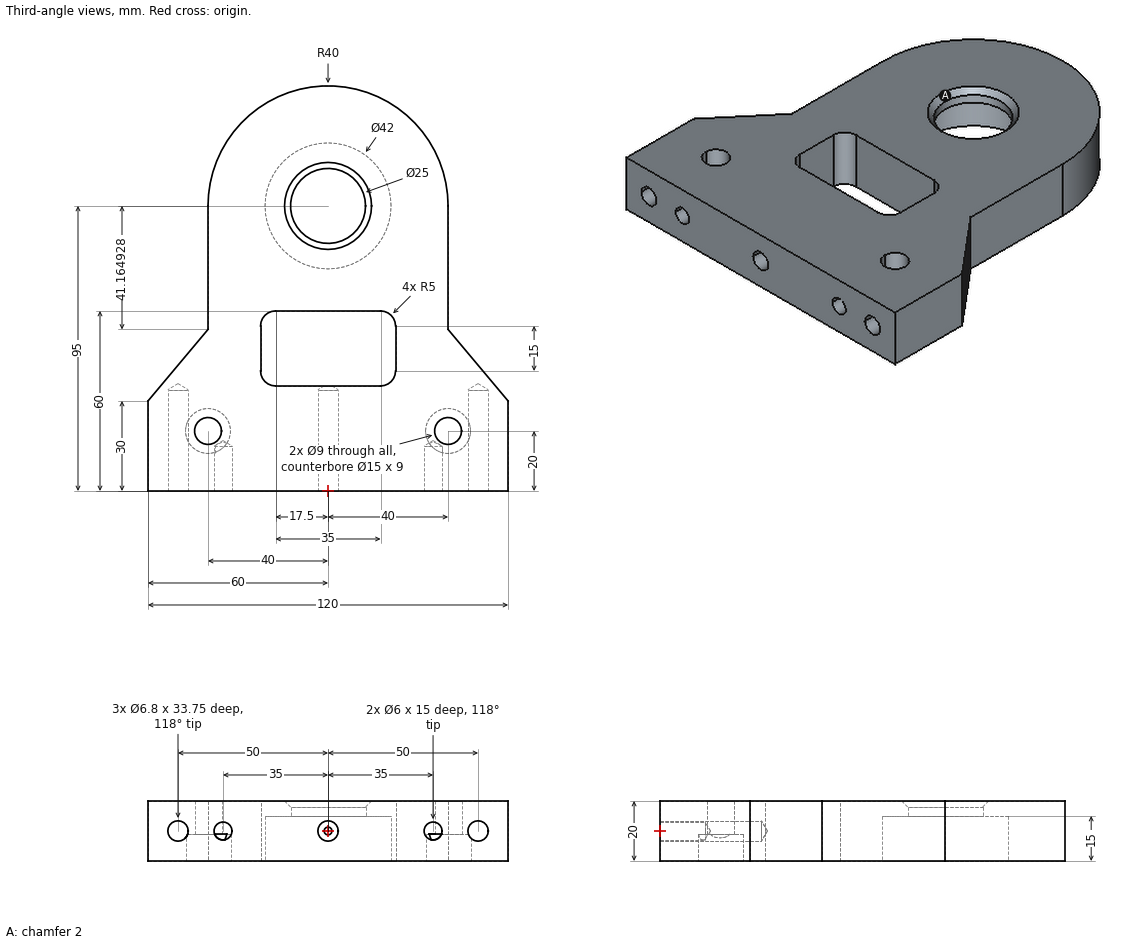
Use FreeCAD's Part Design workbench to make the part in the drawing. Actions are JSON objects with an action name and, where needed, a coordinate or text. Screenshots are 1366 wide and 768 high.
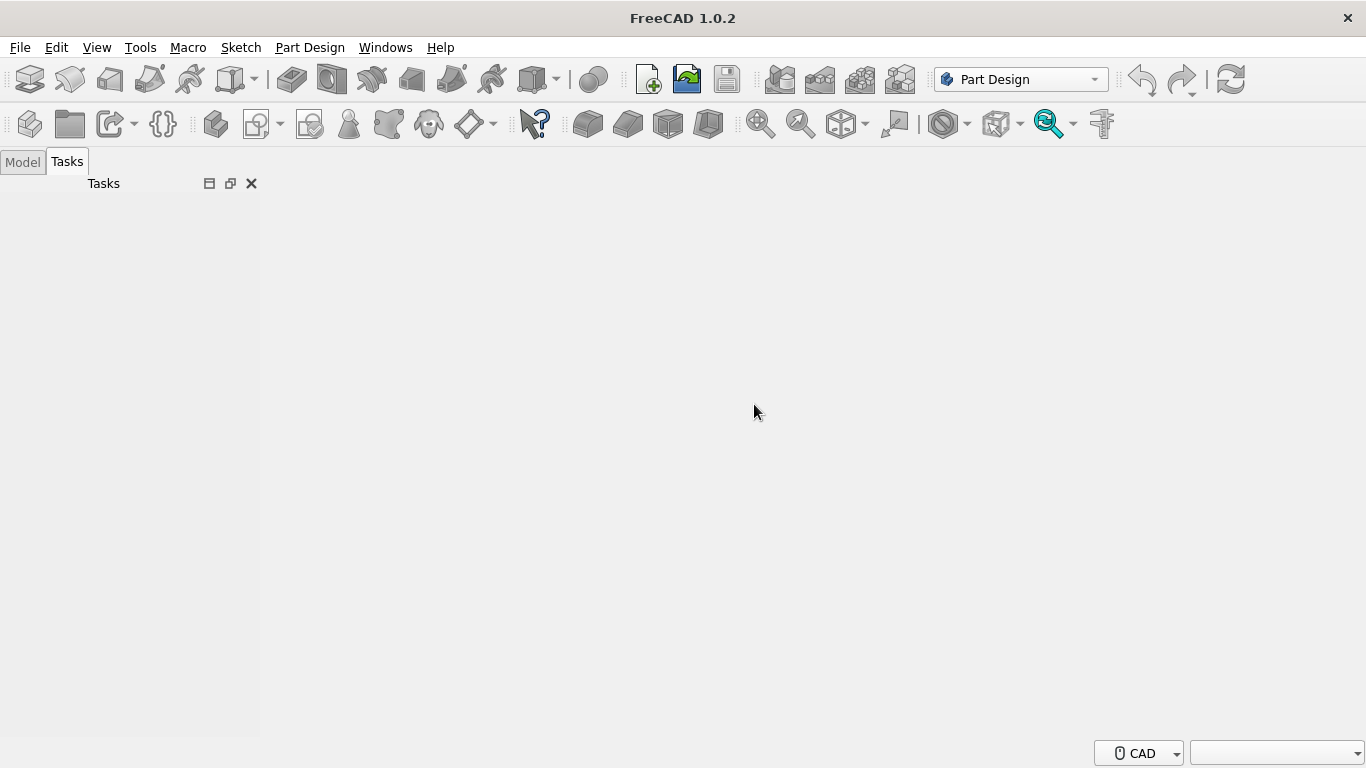
{"action": "left_click", "coordinate": [648, 80]}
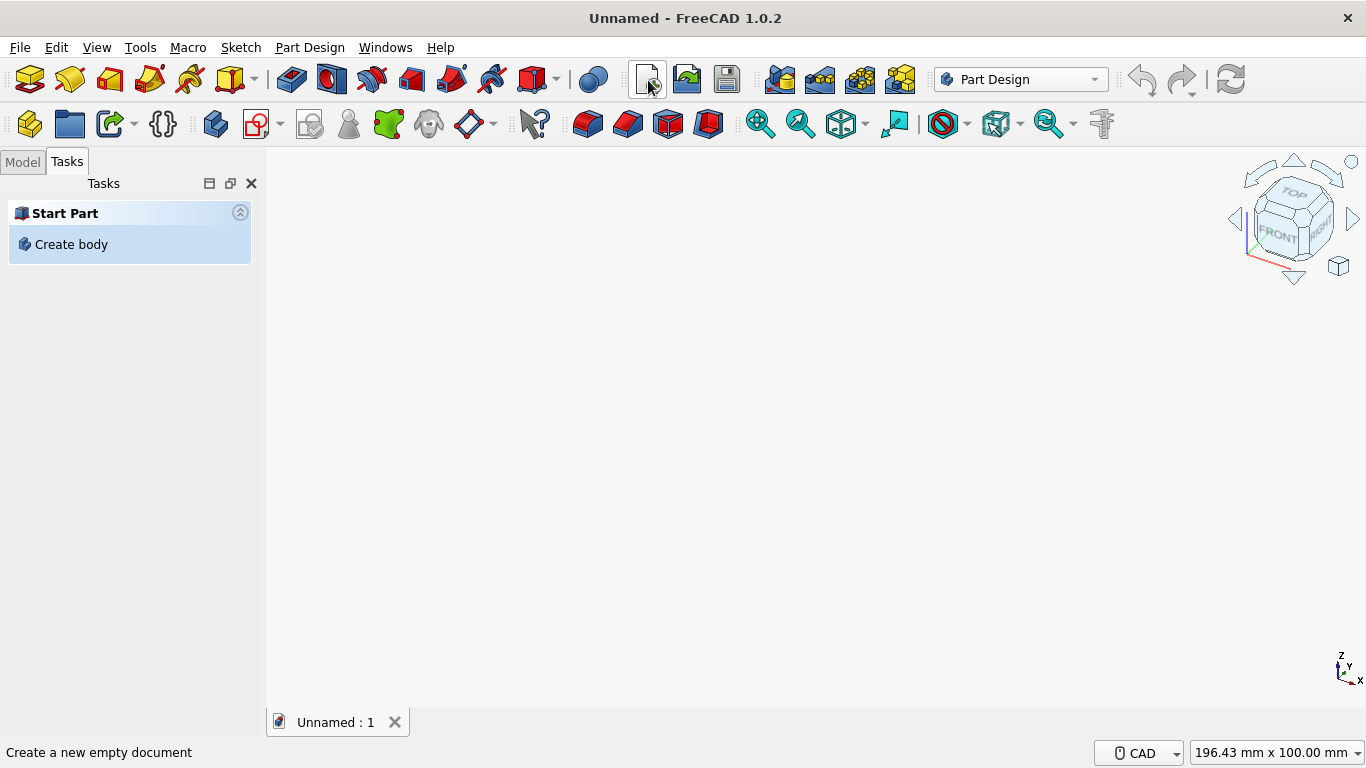
{"action": "left_click", "coordinate": [256, 124]}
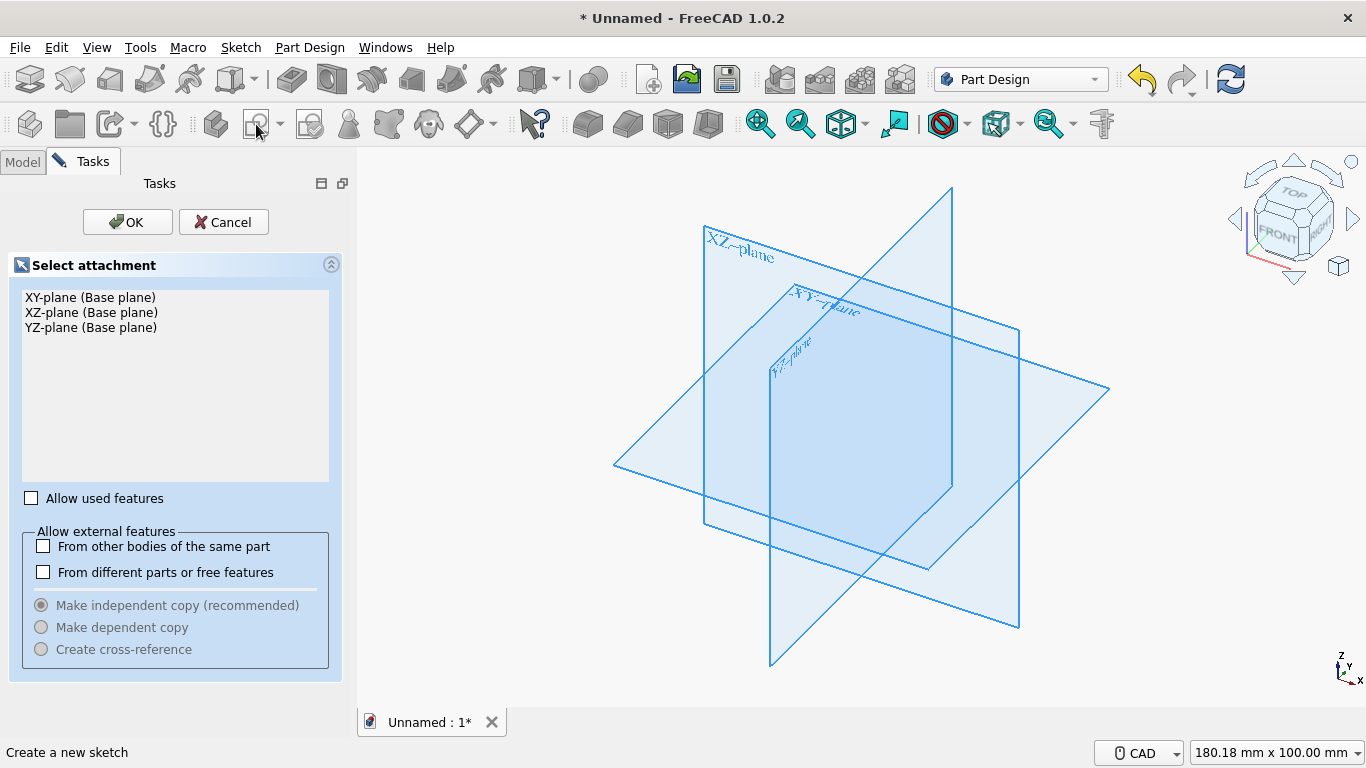
{"action": "left_click", "coordinate": [82, 298]}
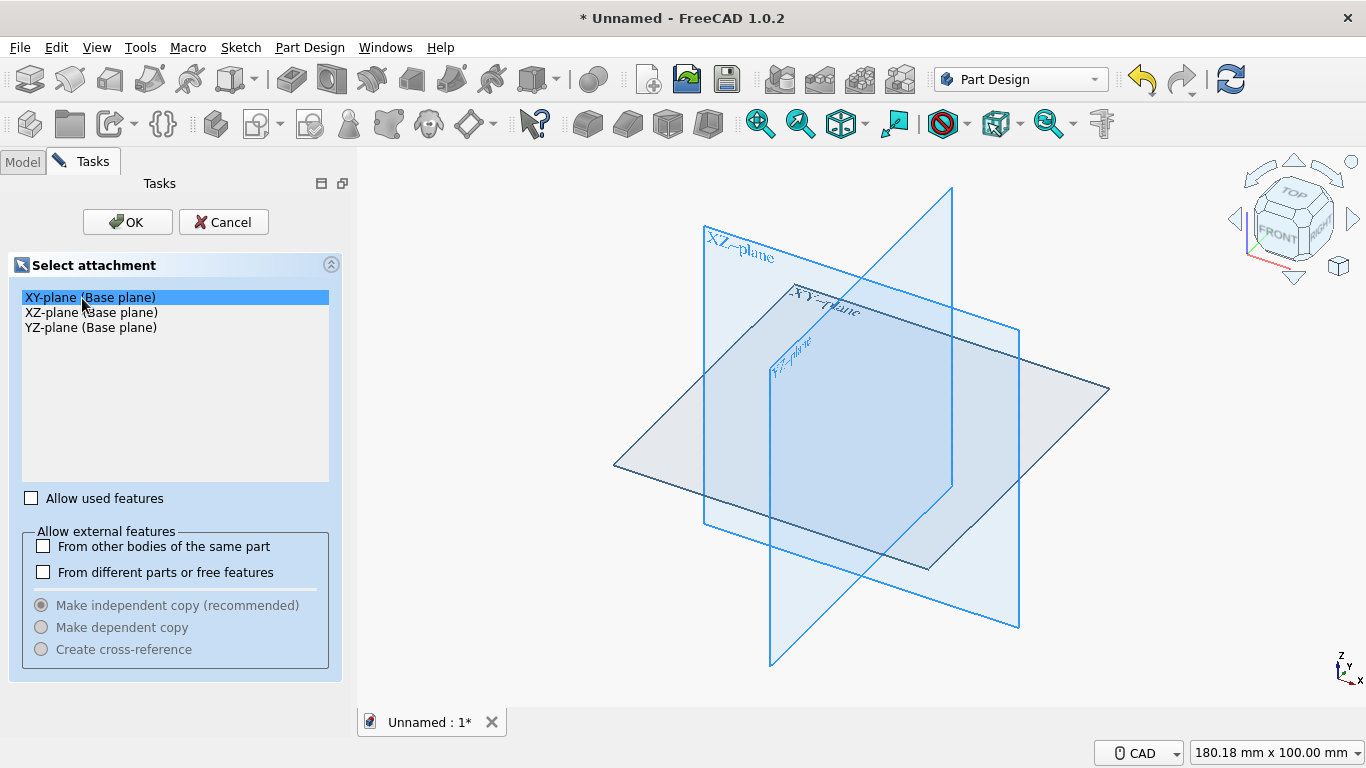
{"action": "left_click", "coordinate": [128, 222]}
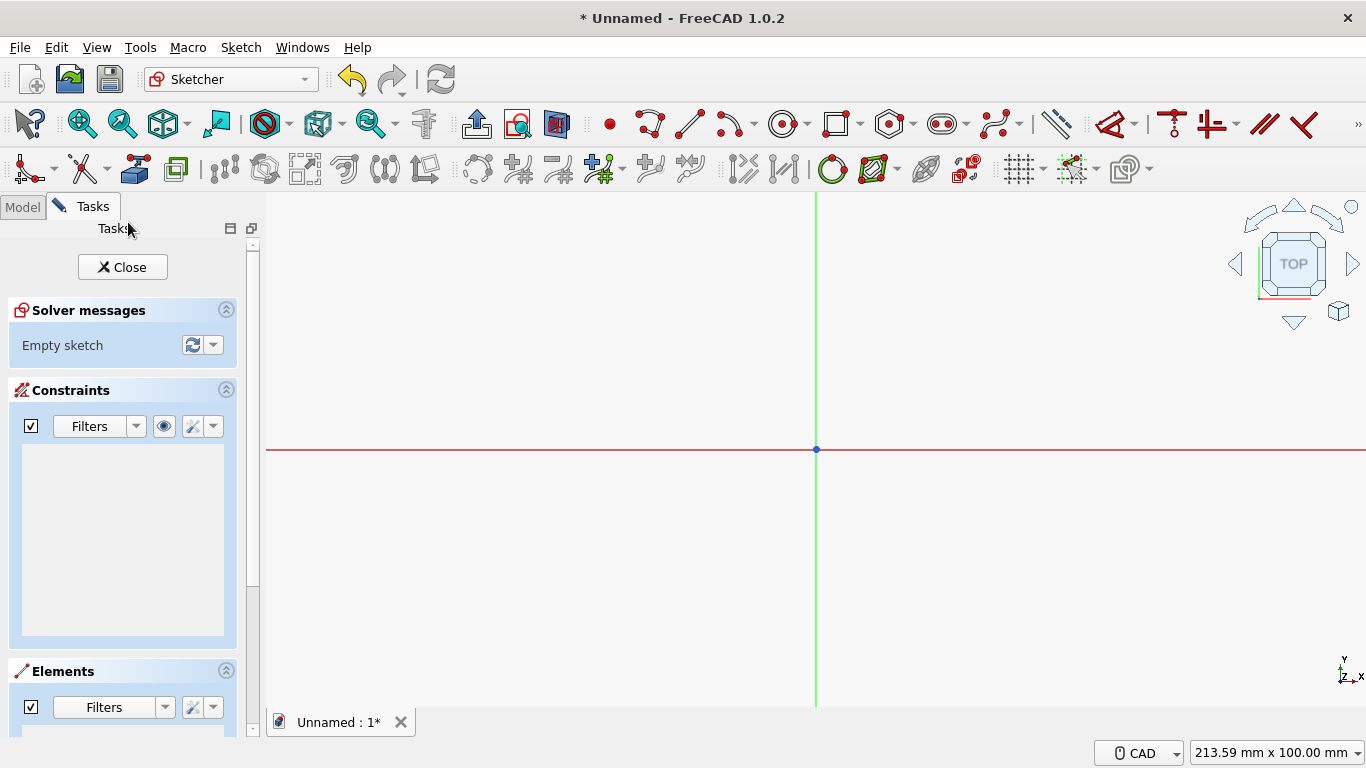
{"action": "scroll", "coordinate": [692, 679], "scroll_direction": "down", "scroll_amount": 4}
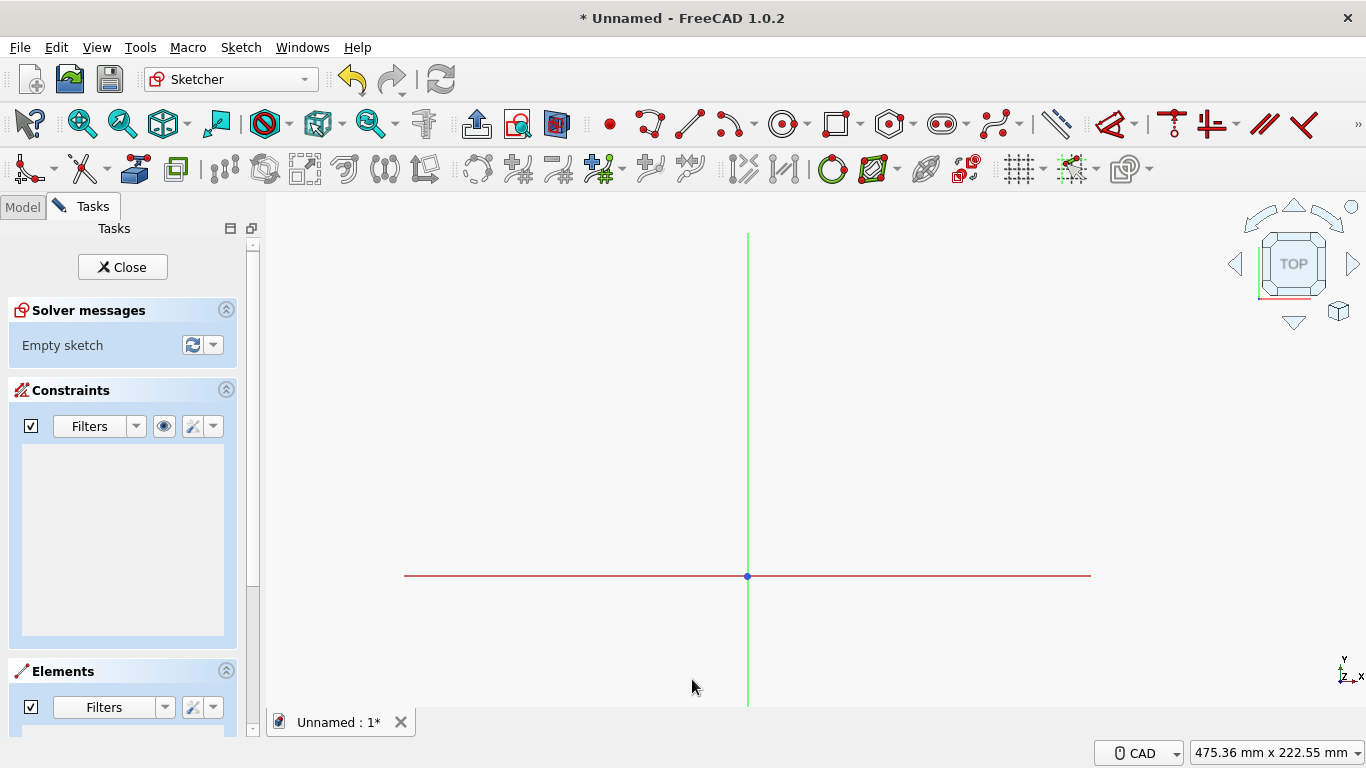
{"action": "left_click", "coordinate": [650, 124]}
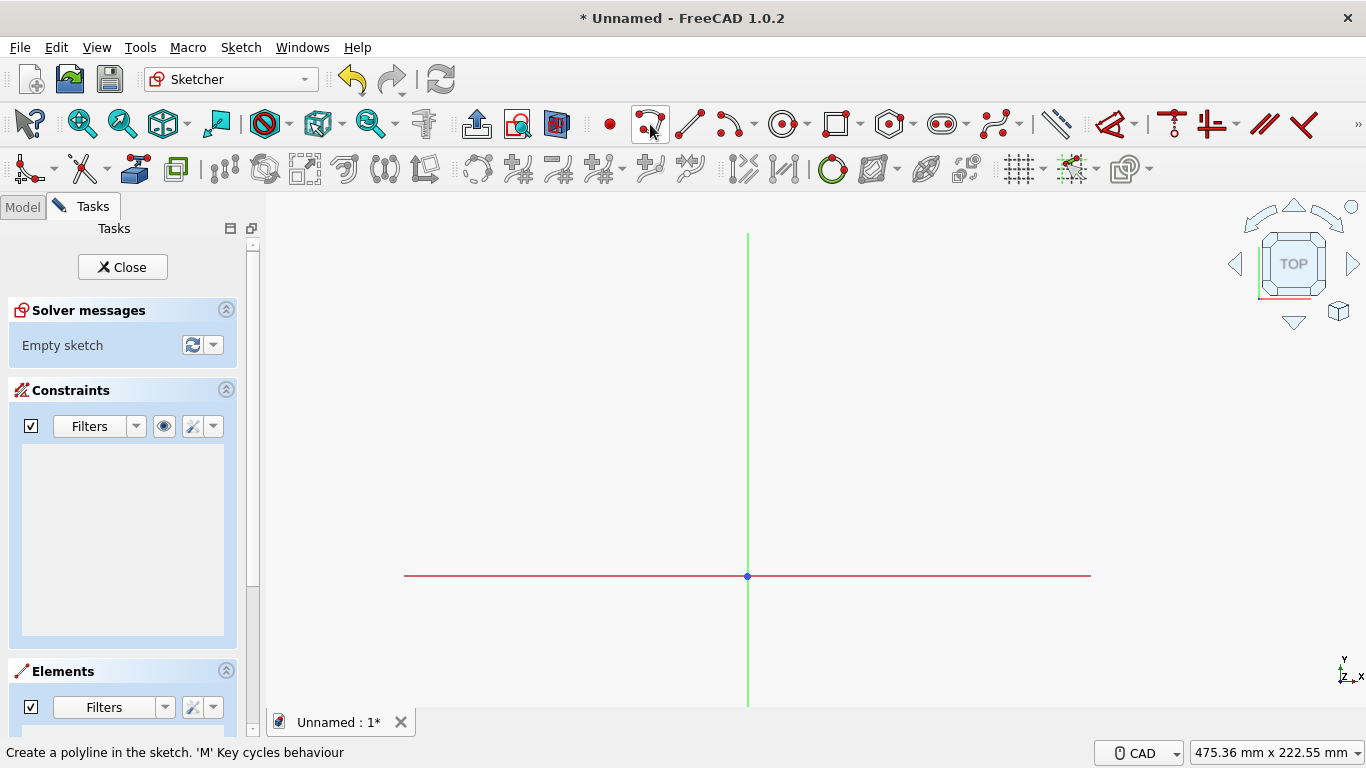
{"action": "left_click", "coordinate": [655, 357]}
{"action": "left_click", "coordinate": [655, 452]}
{"action": "left_click", "coordinate": [609, 507]}
{"action": "left_click", "coordinate": [609, 576]}
{"action": "left_click", "coordinate": [887, 567]}
{"action": "left_click", "coordinate": [887, 507]}
{"action": "left_click", "coordinate": [840, 452]}
{"action": "left_click", "coordinate": [840, 357]}
{"action": "right_click", "coordinate": [840, 357]}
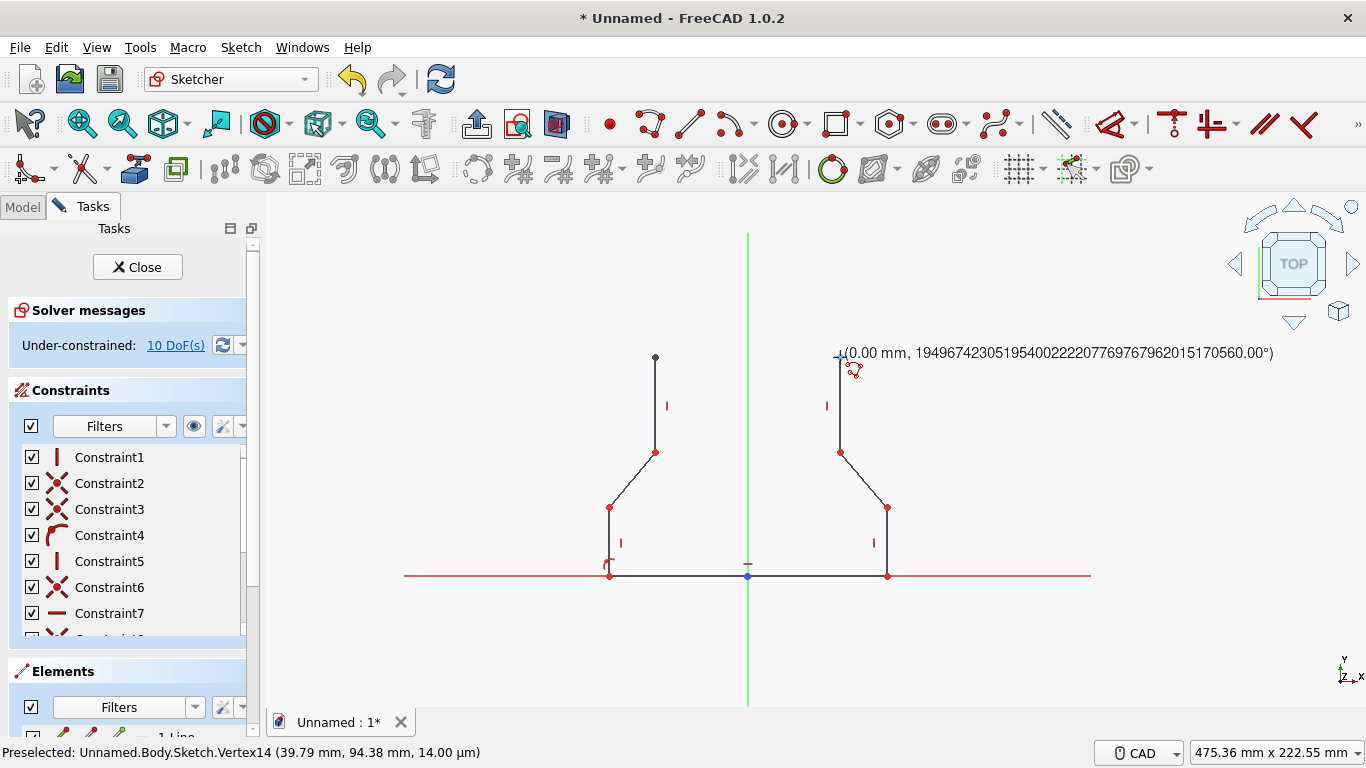
{"action": "key", "text": "g 3 a"}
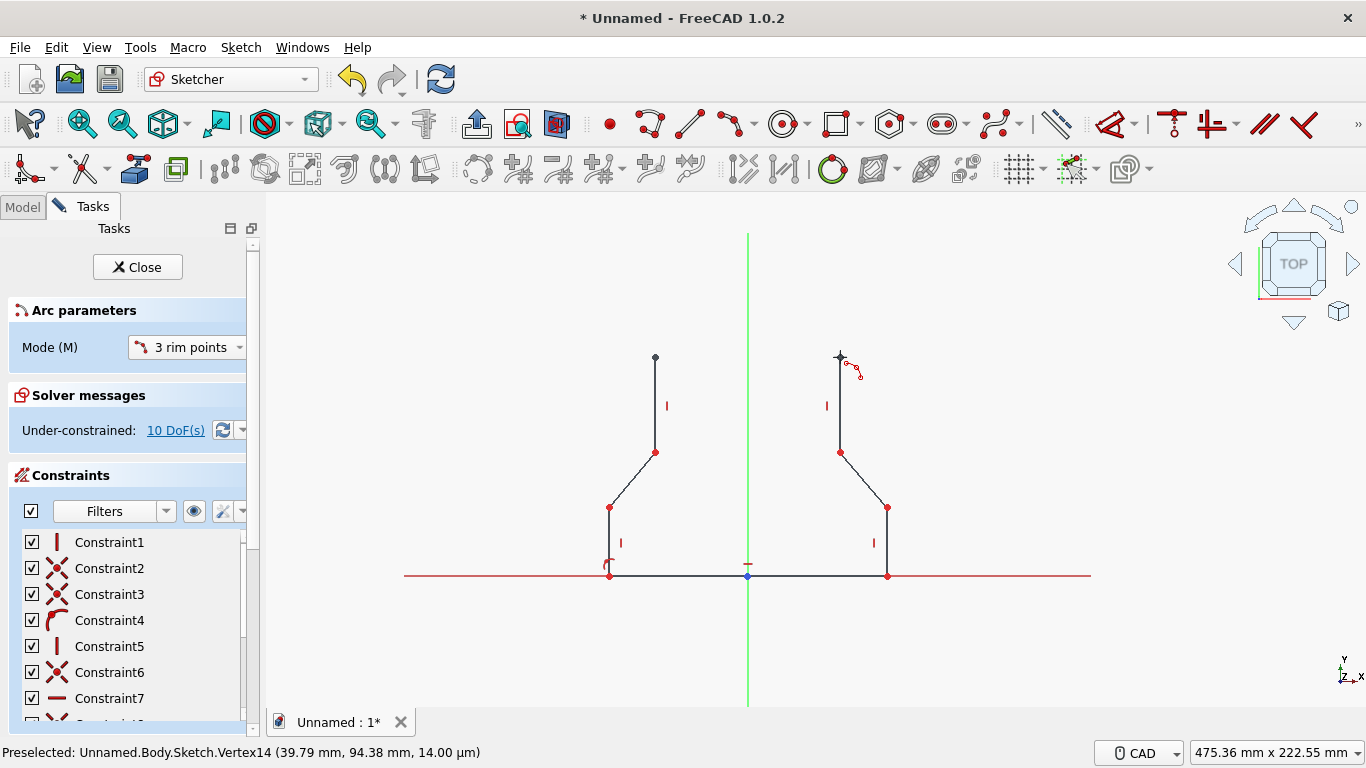
{"action": "left_click", "coordinate": [840, 358]}
{"action": "left_click", "coordinate": [655, 358]}
{"action": "left_click", "coordinate": [777, 269]}